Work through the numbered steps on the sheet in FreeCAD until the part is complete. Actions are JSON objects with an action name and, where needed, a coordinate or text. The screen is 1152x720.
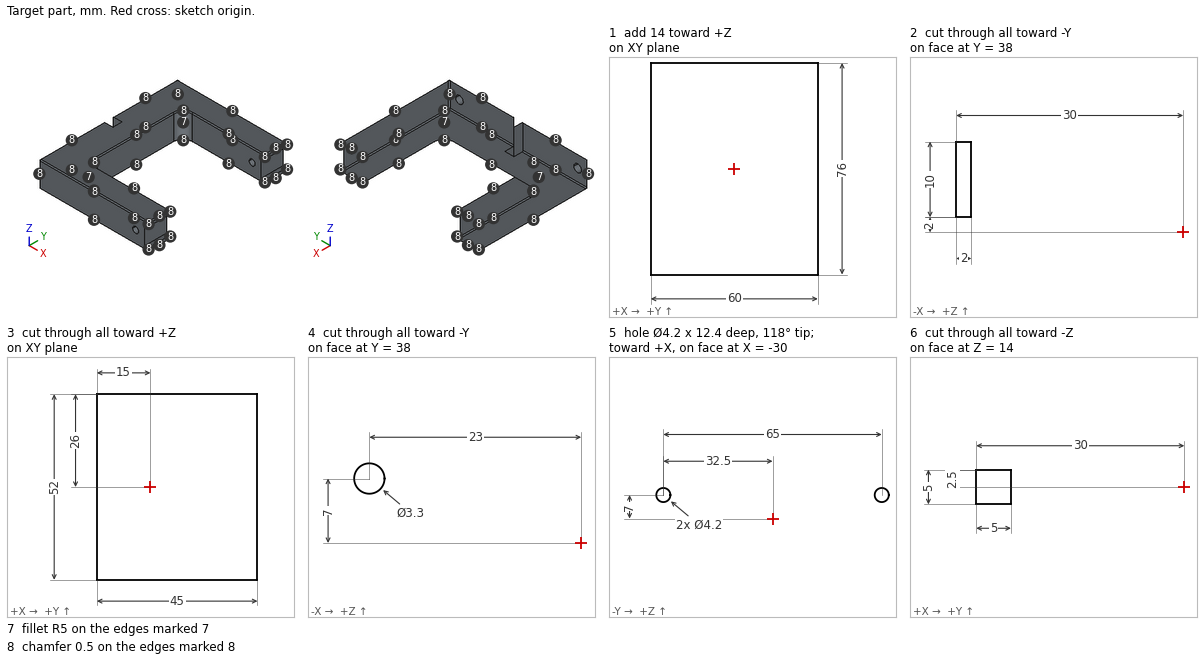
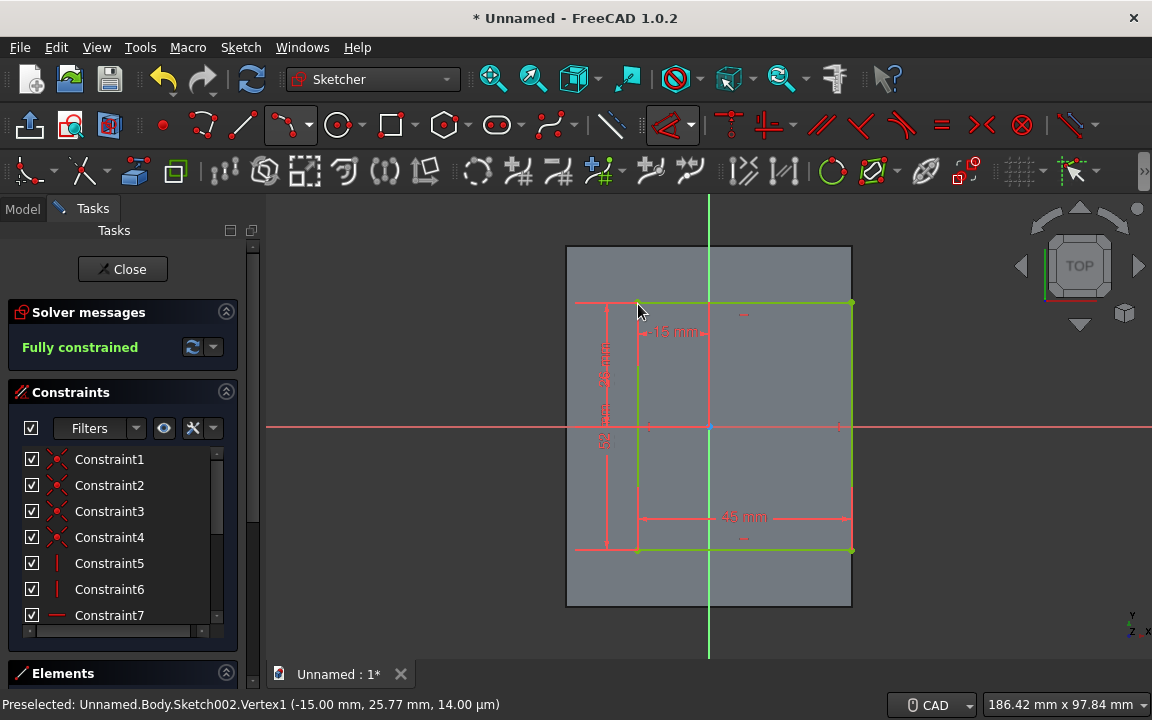
{"action": "left_click", "coordinate": [123, 269]}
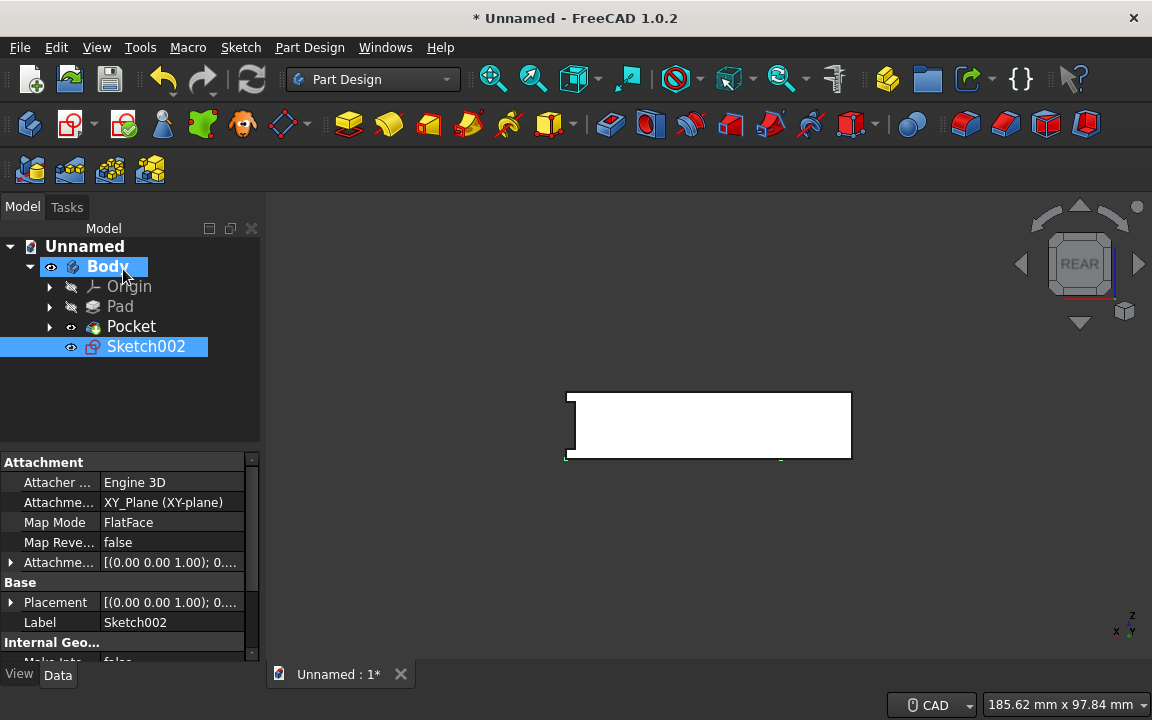
{"action": "left_click", "coordinate": [612, 124]}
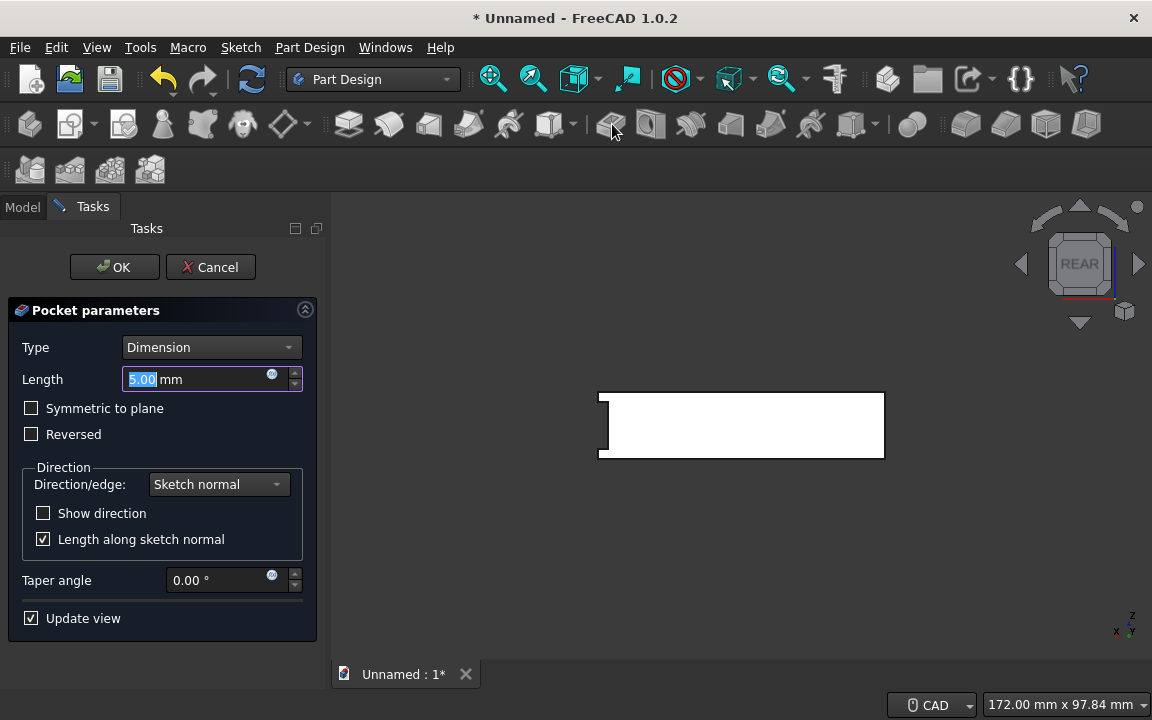
{"action": "left_click", "coordinate": [212, 348]}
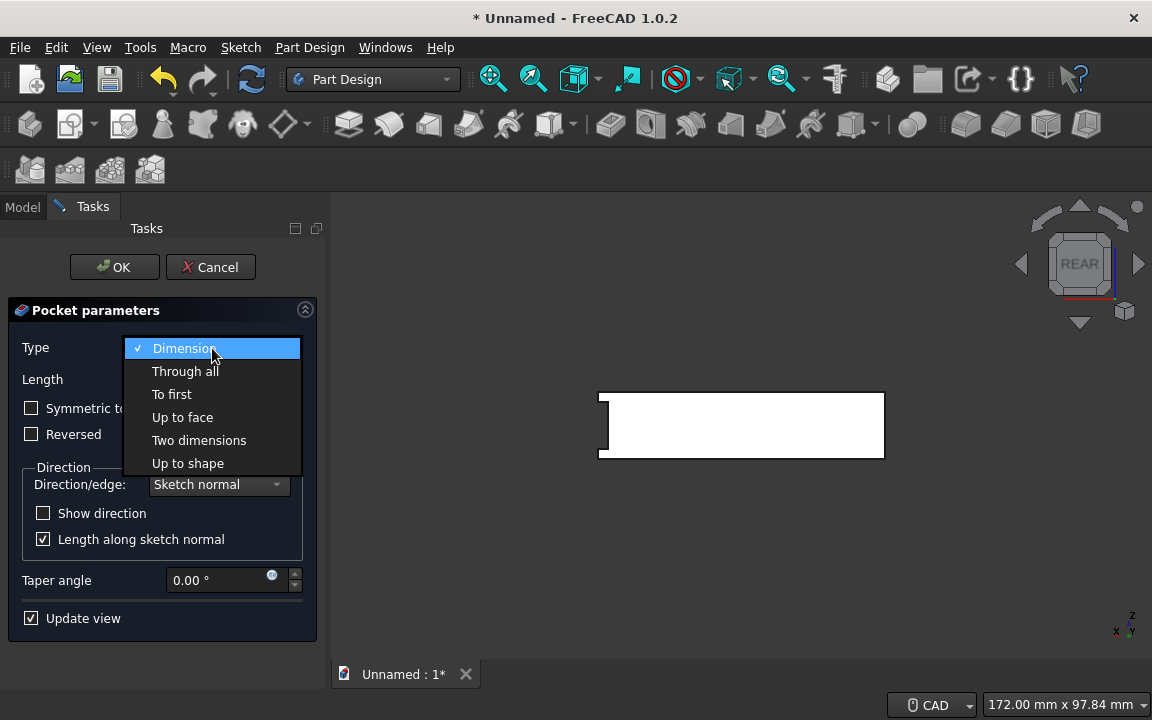
{"action": "left_click", "coordinate": [212, 372]}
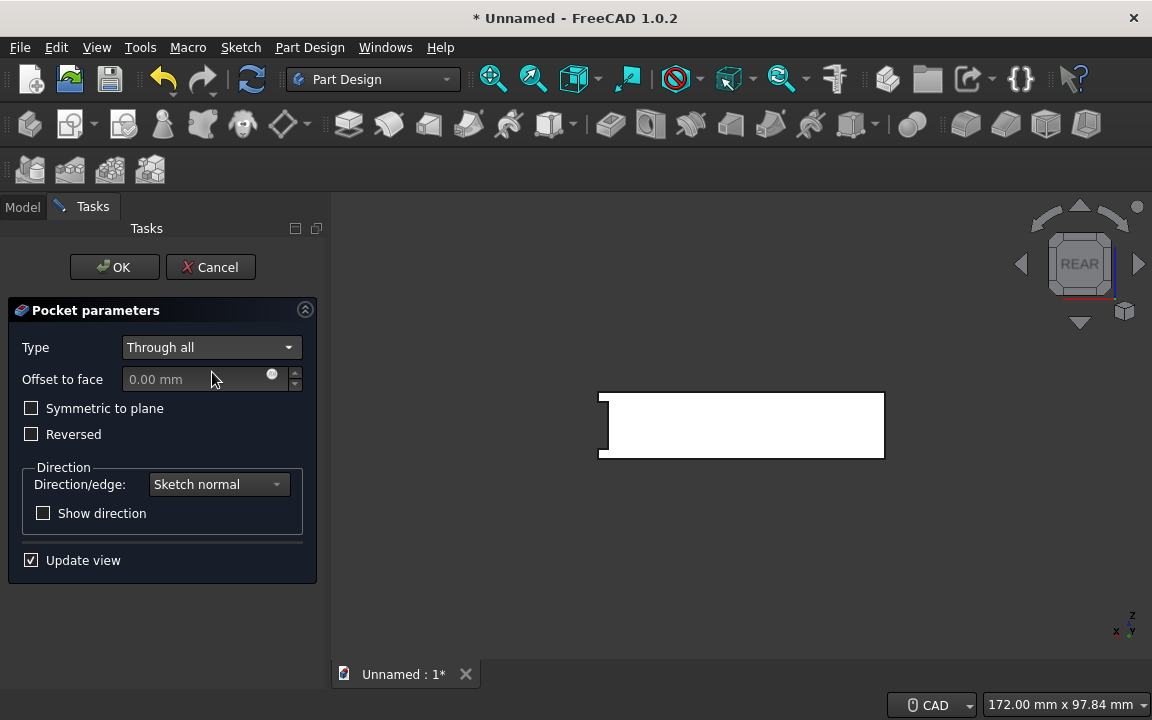
{"action": "left_click", "coordinate": [30, 434]}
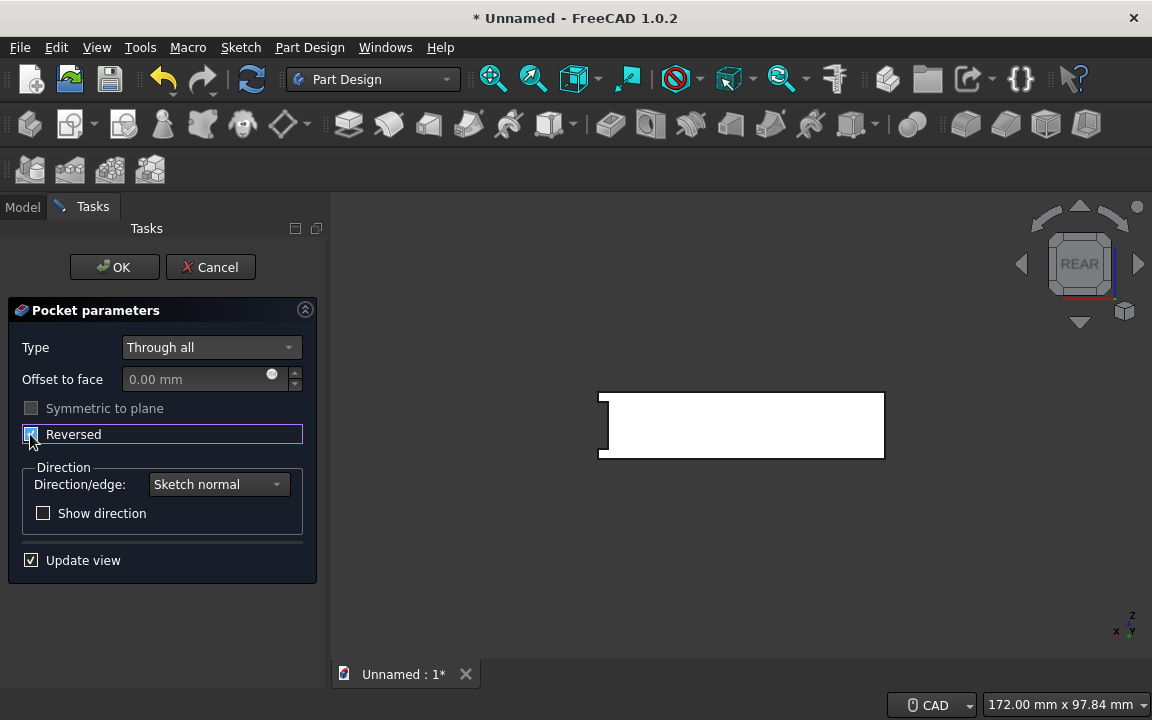
{"action": "left_click", "coordinate": [115, 267]}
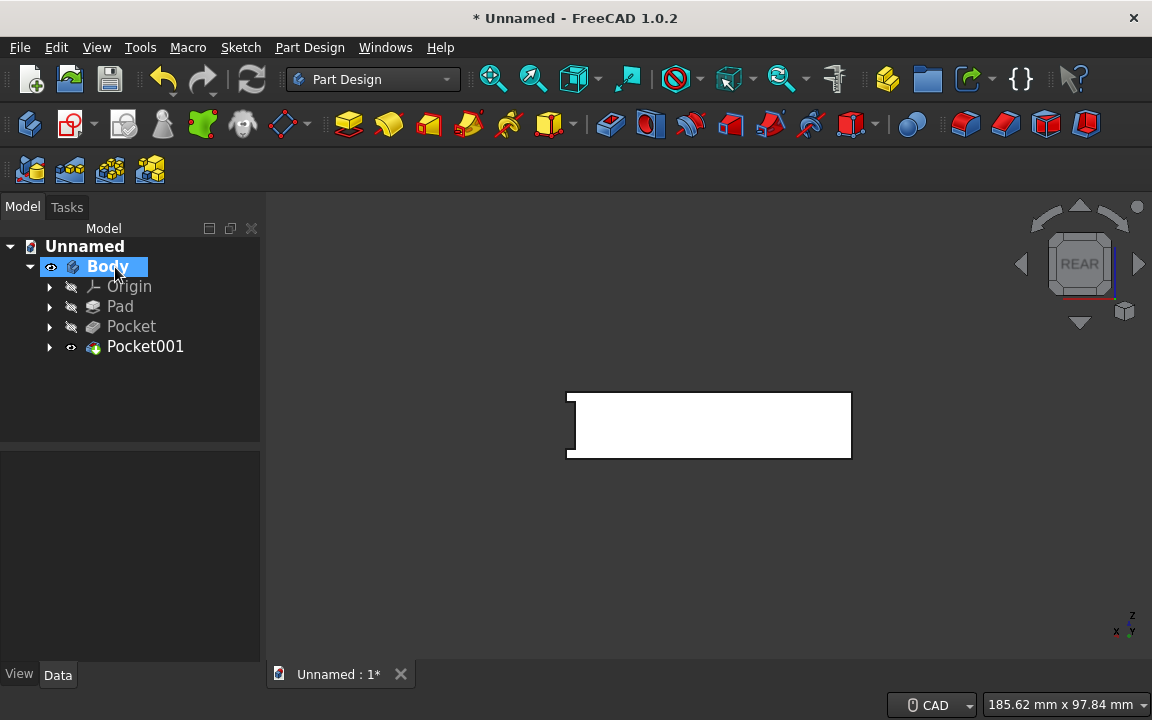
{"action": "key", "text": "v f"}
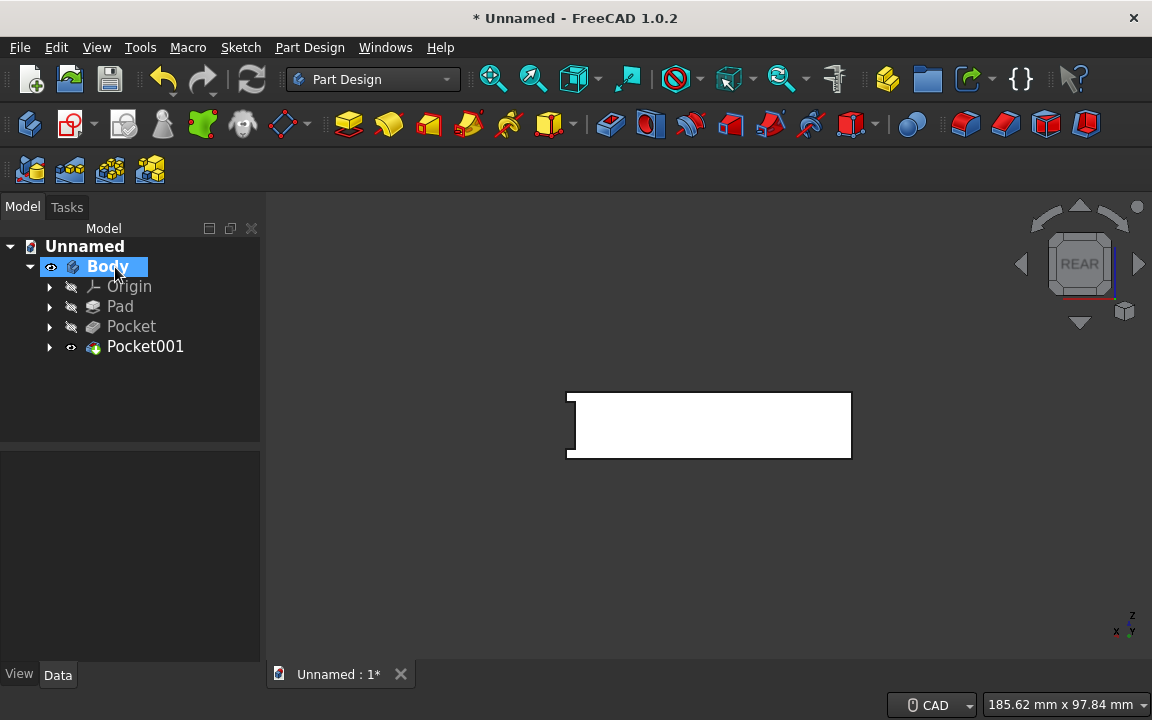
{"action": "left_click", "coordinate": [627, 424]}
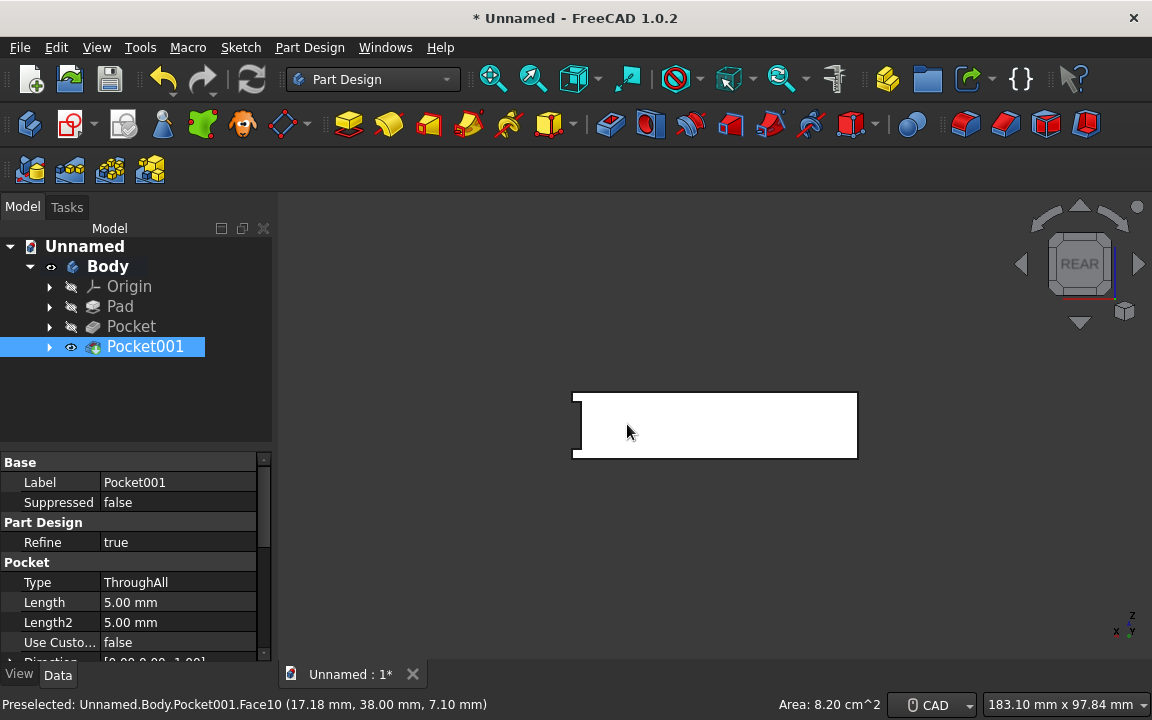
{"action": "left_click", "coordinate": [70, 124]}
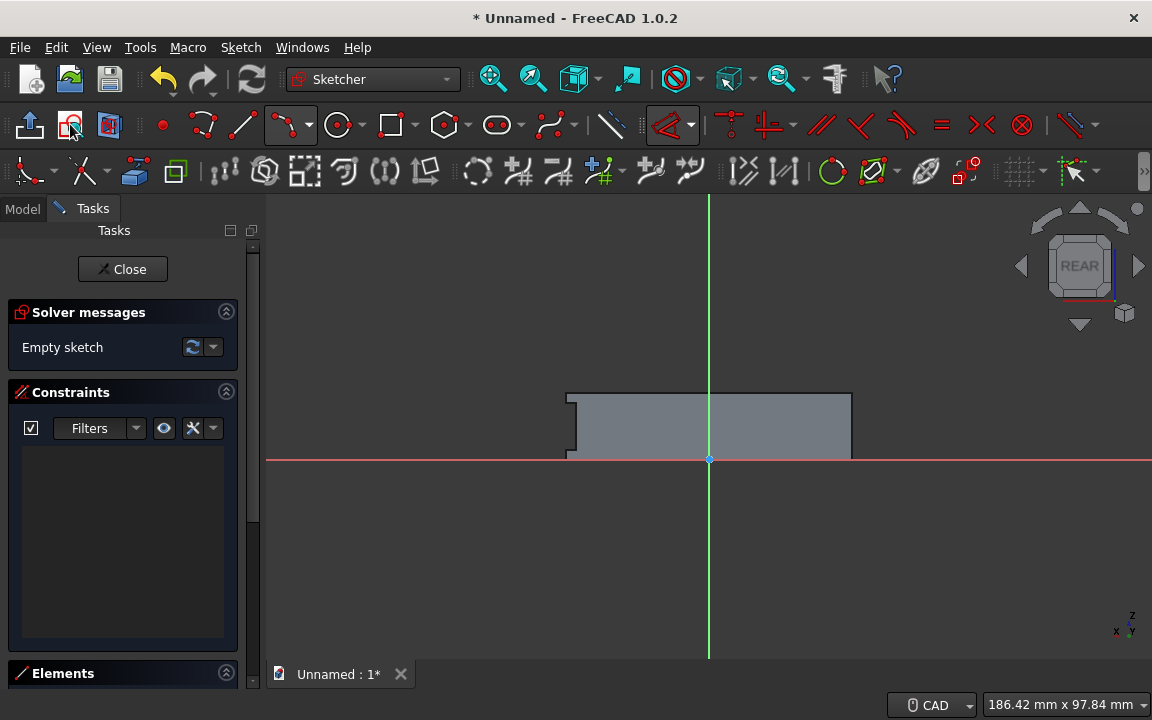
{"action": "scroll", "coordinate": [598, 426], "scroll_direction": "up", "scroll_amount": 15}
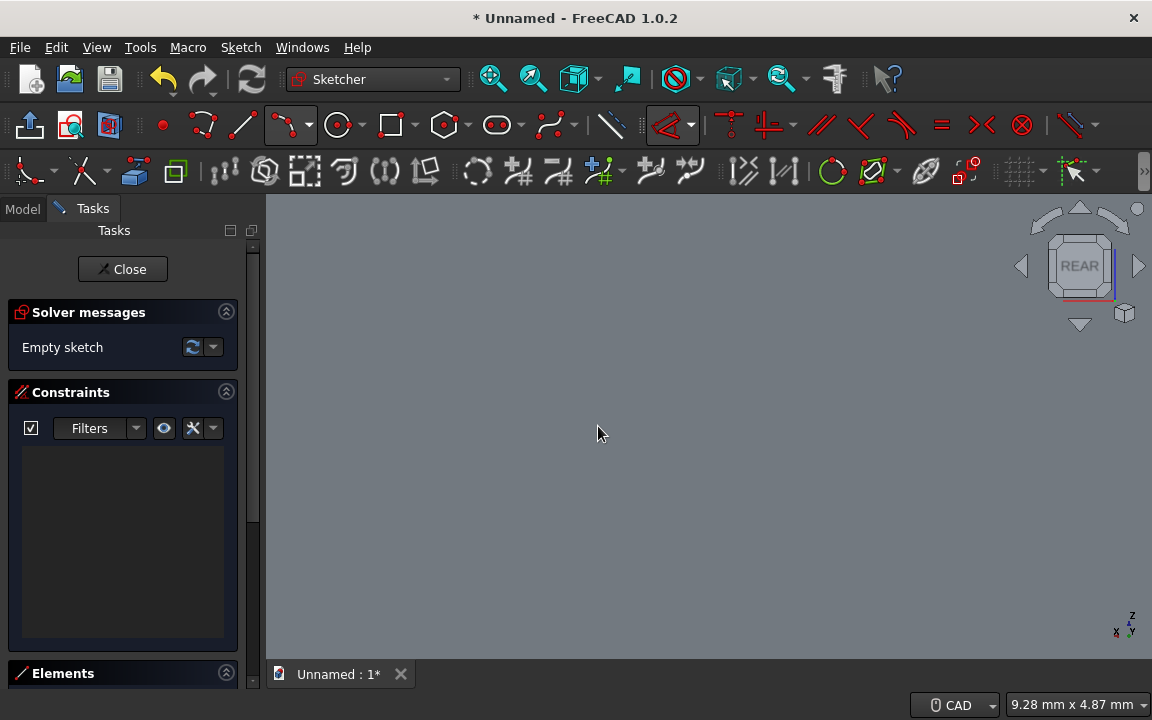
{"action": "left_click", "coordinate": [338, 126]}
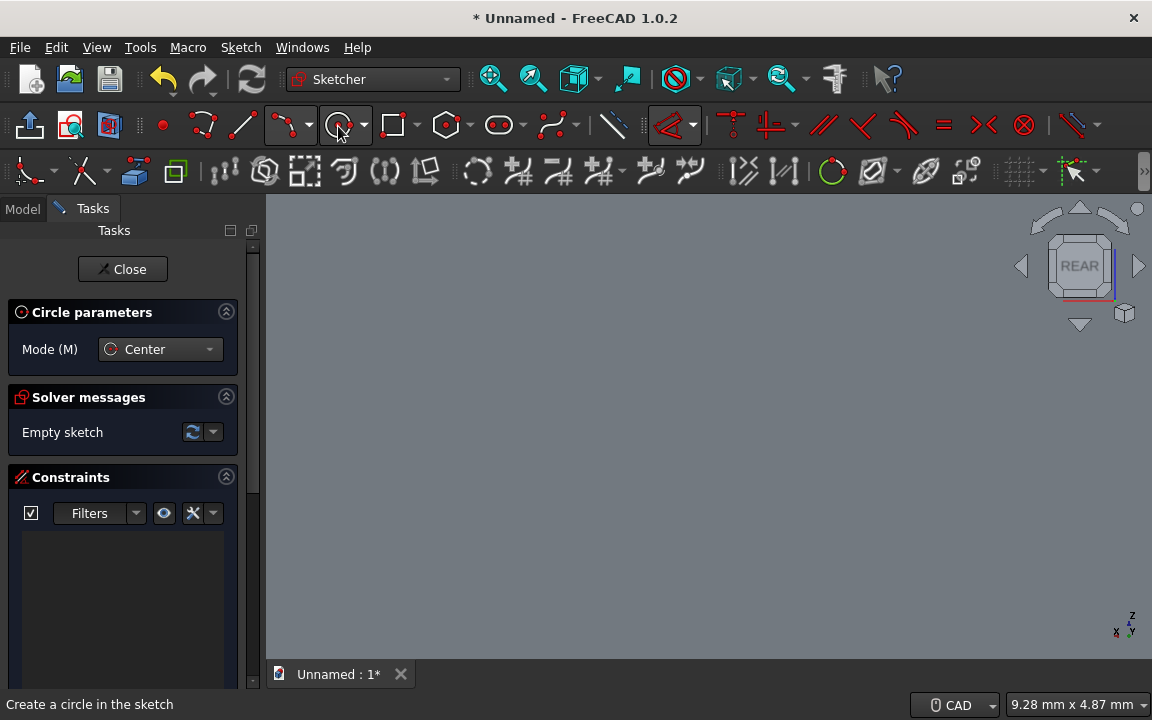
{"action": "left_click", "coordinate": [625, 426]}
{"action": "left_click", "coordinate": [736, 315]}
{"action": "key", "text": "Escape"}